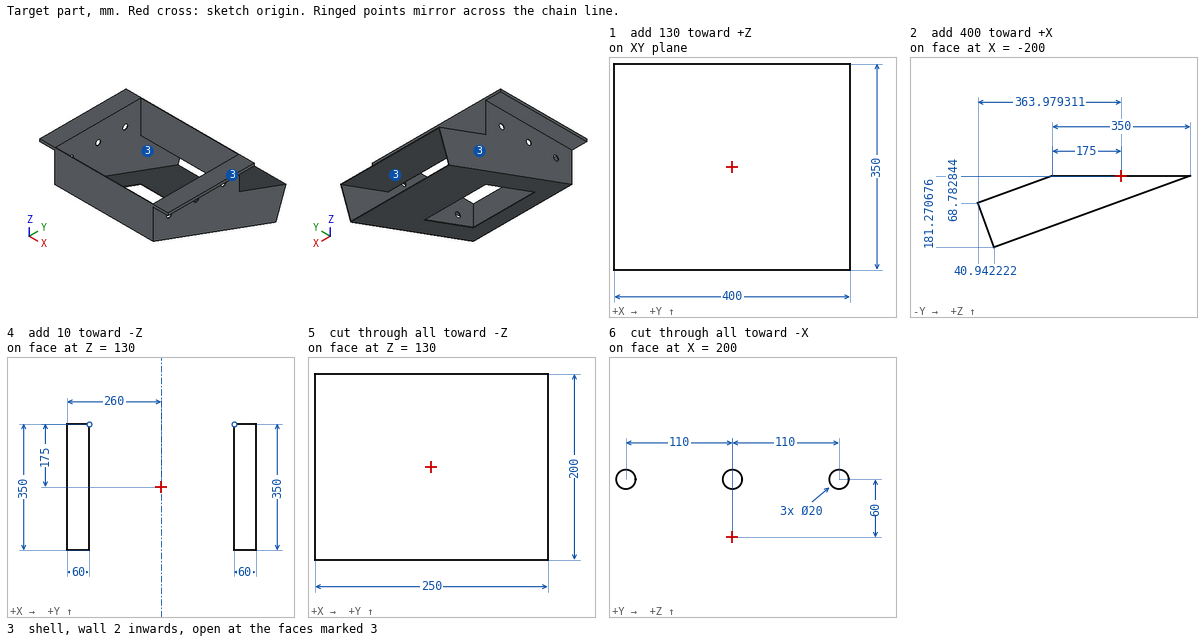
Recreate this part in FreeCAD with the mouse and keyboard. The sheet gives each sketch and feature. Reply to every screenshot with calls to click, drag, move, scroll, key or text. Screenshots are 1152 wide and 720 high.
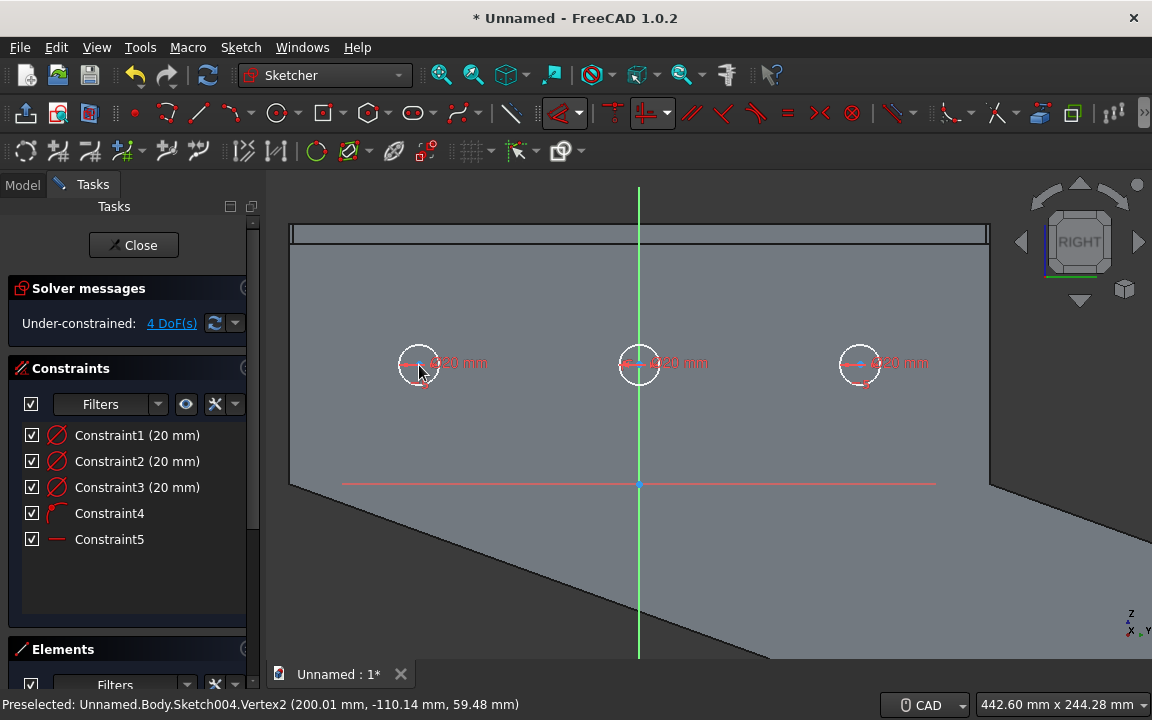
click(860, 365)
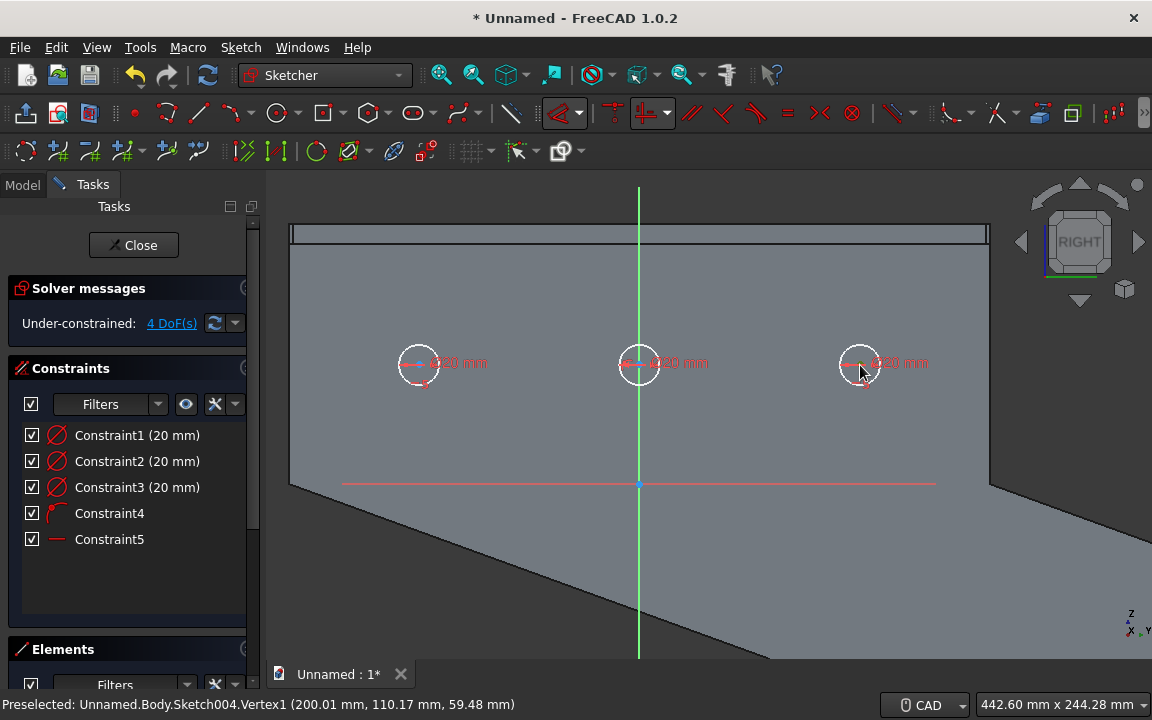
click(639, 365)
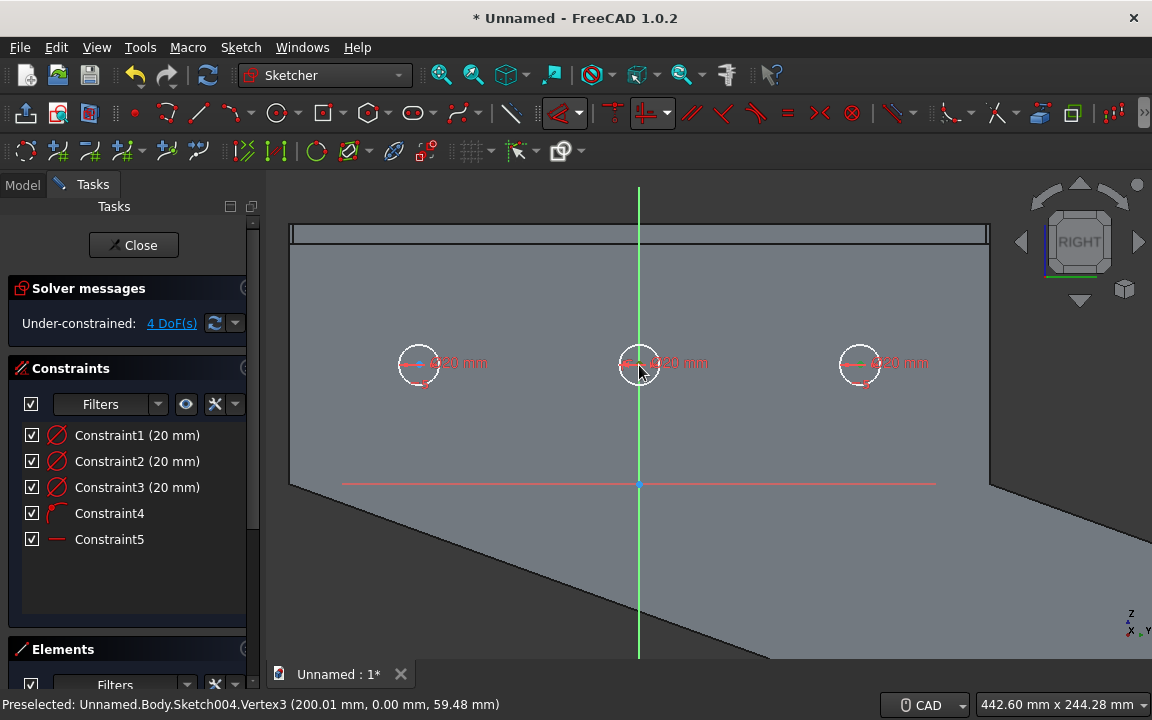
key(h)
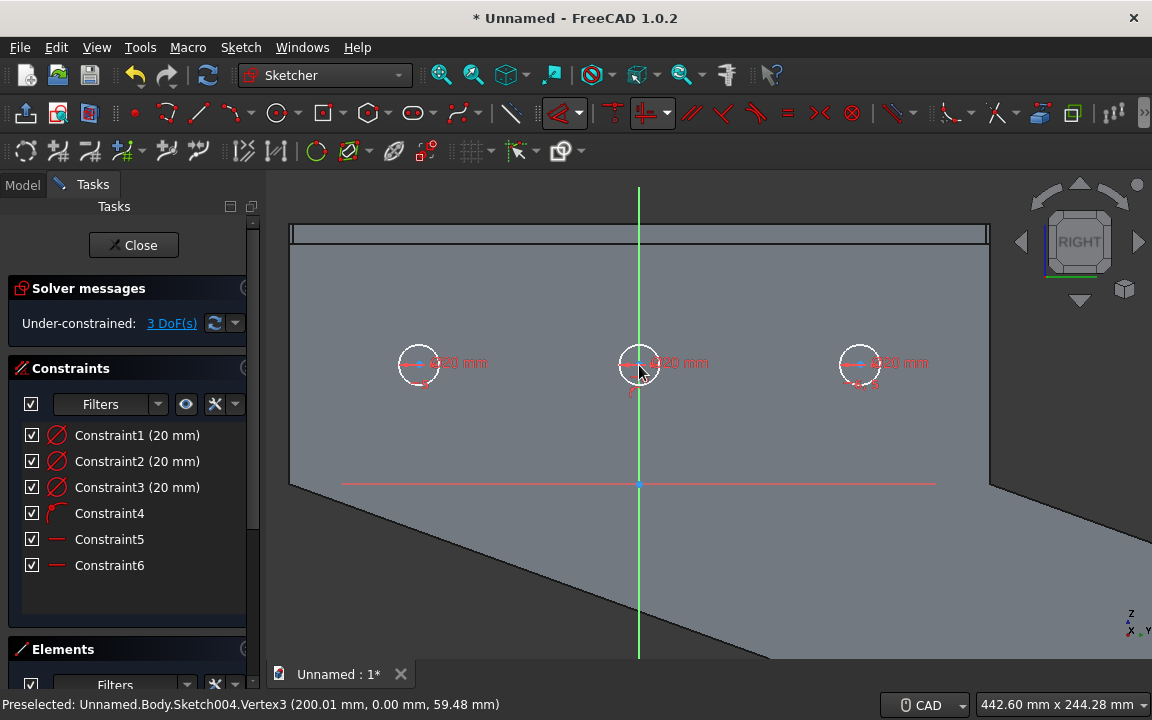
click(860, 365)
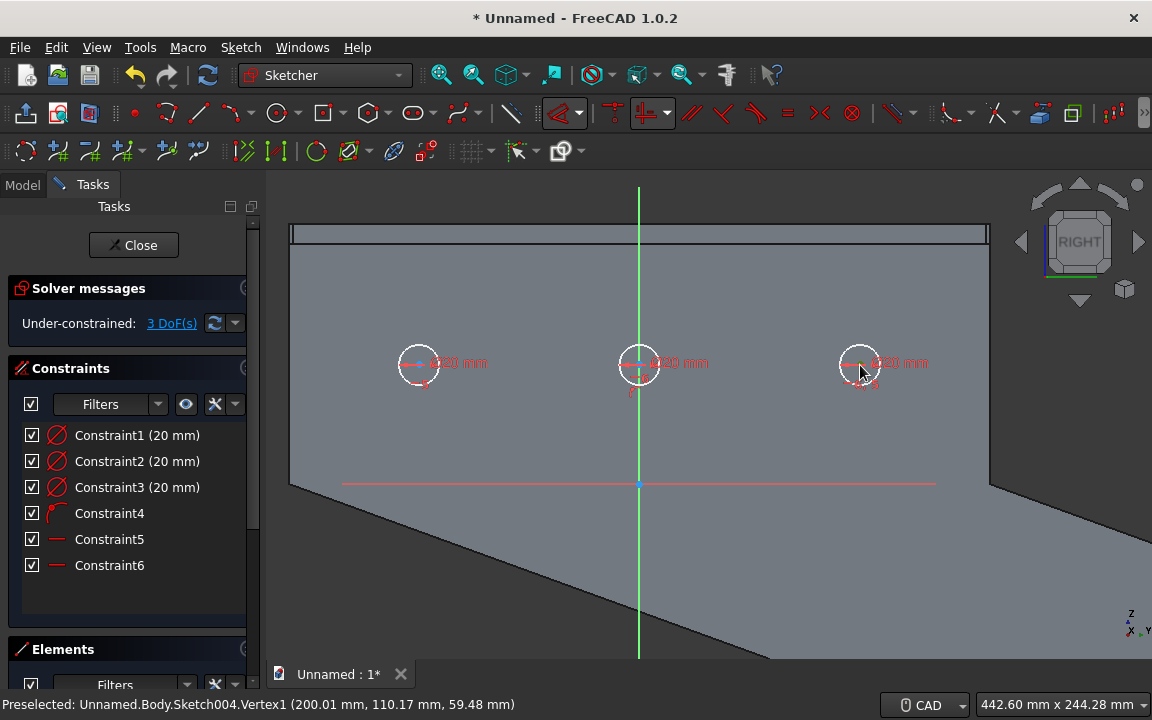
click(582, 114)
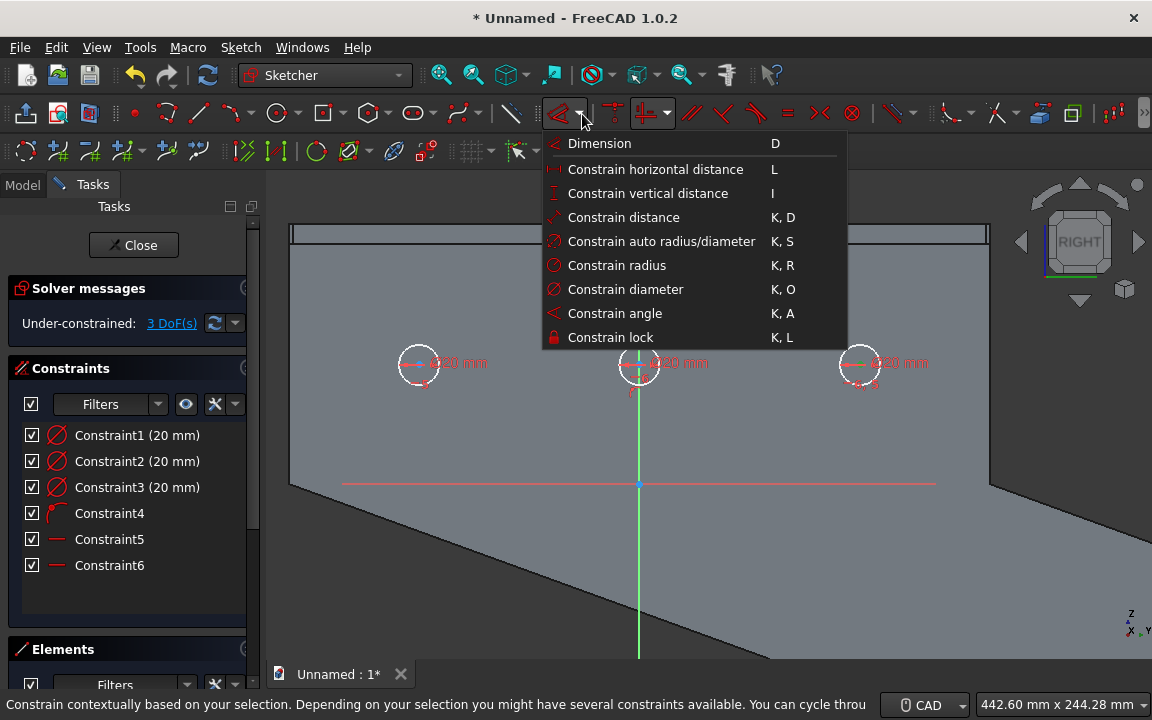
click(695, 193)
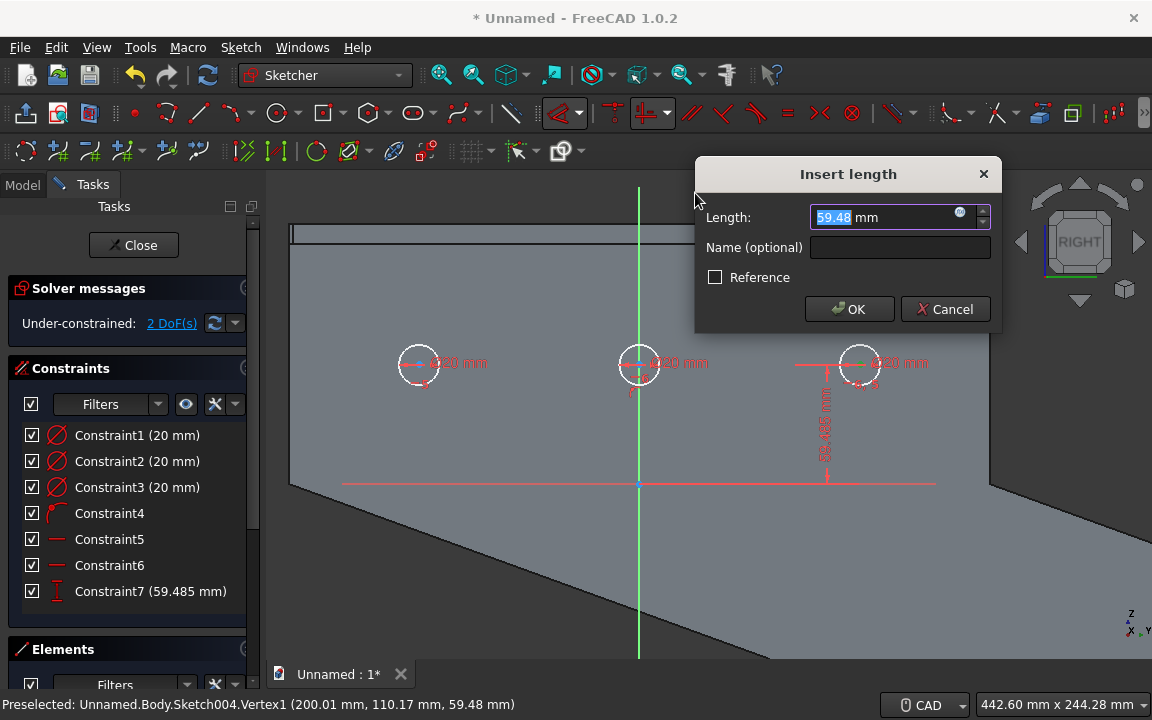
text(60)
key(Return)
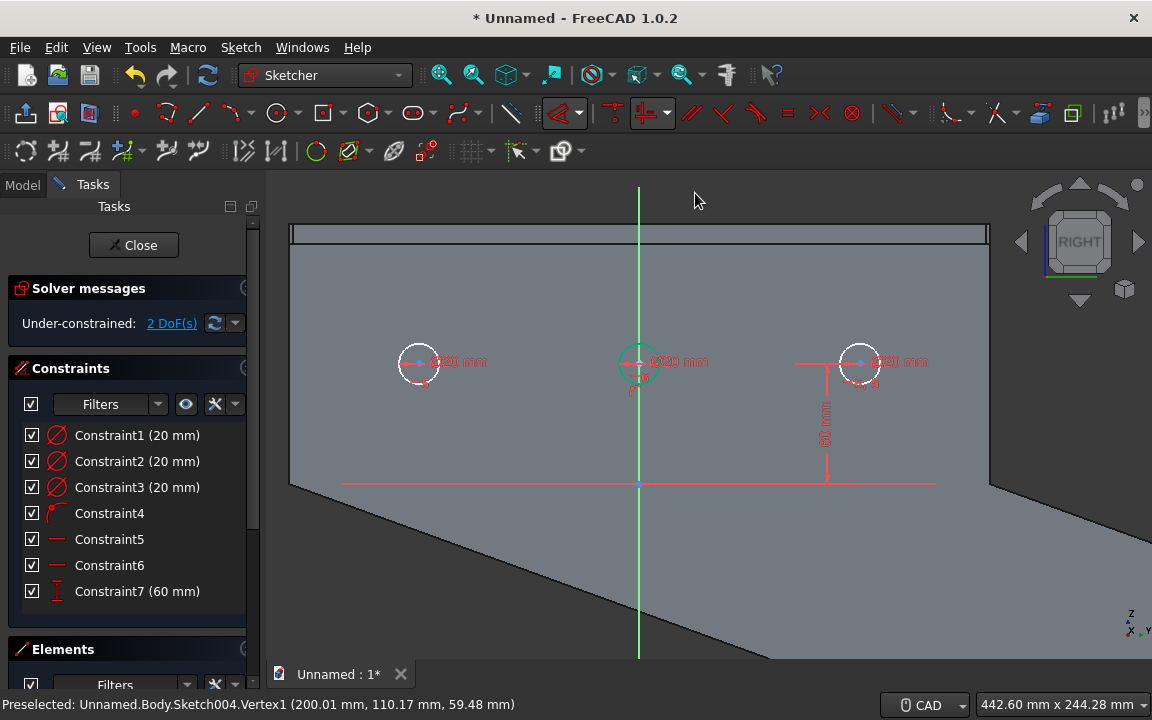
click(860, 364)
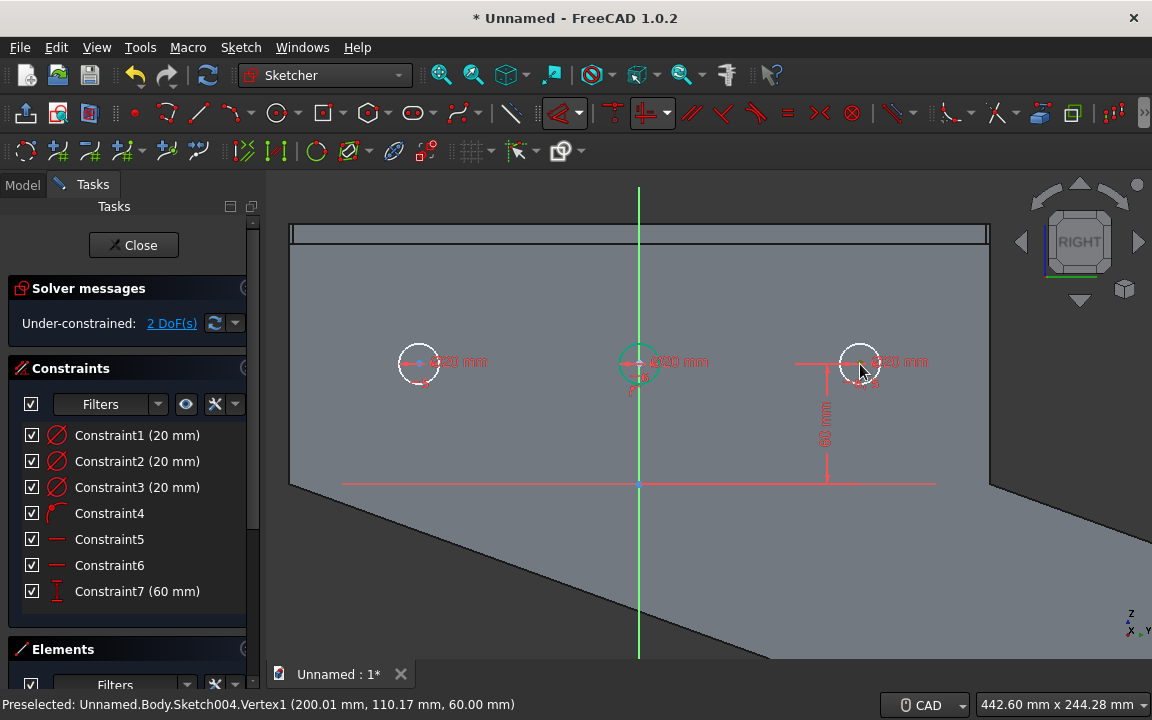
key(l)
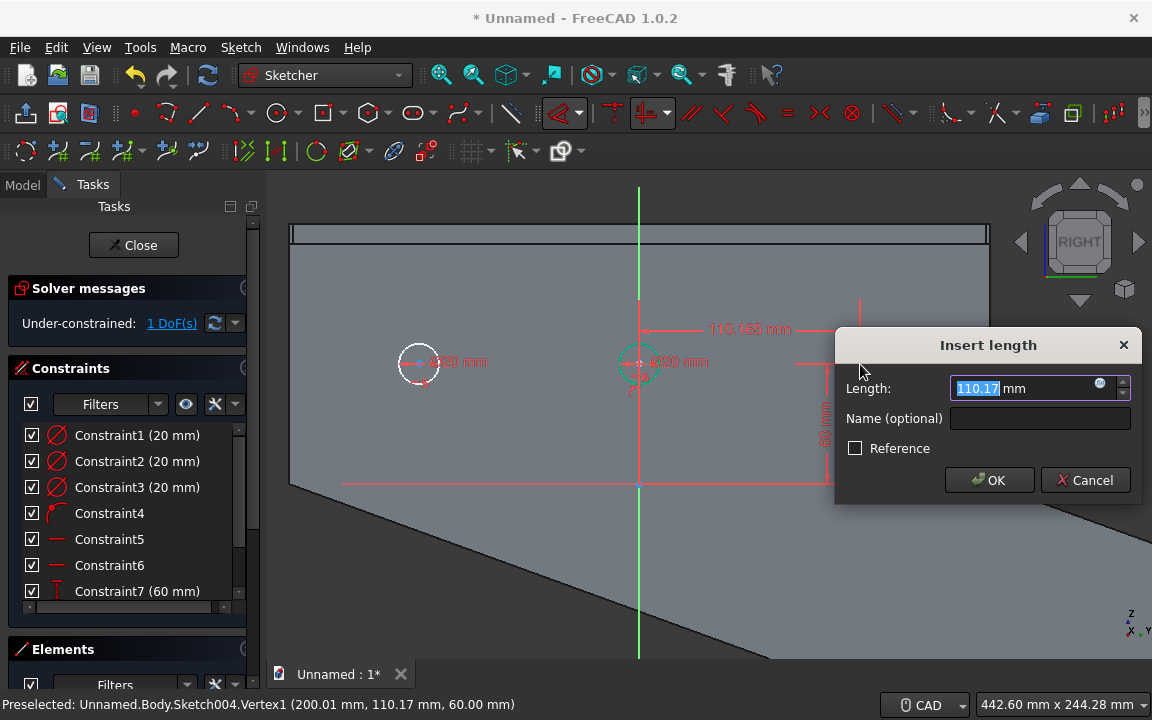
text(110)
key(Return)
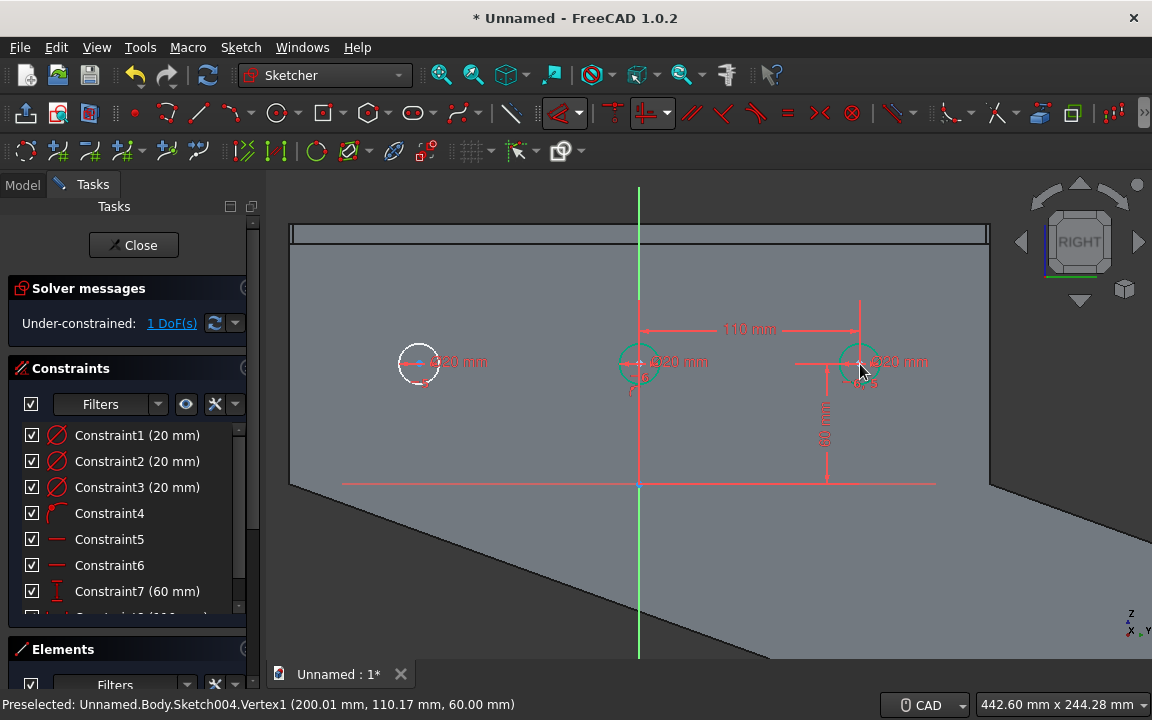
click(419, 364)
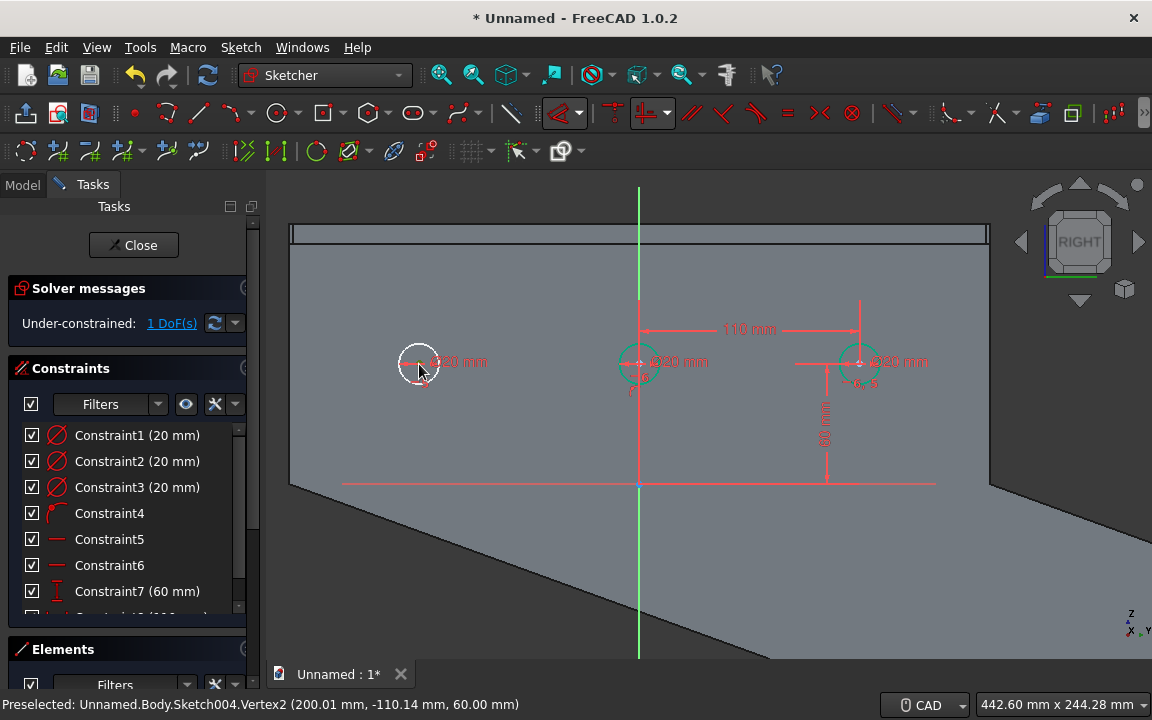
key(l)